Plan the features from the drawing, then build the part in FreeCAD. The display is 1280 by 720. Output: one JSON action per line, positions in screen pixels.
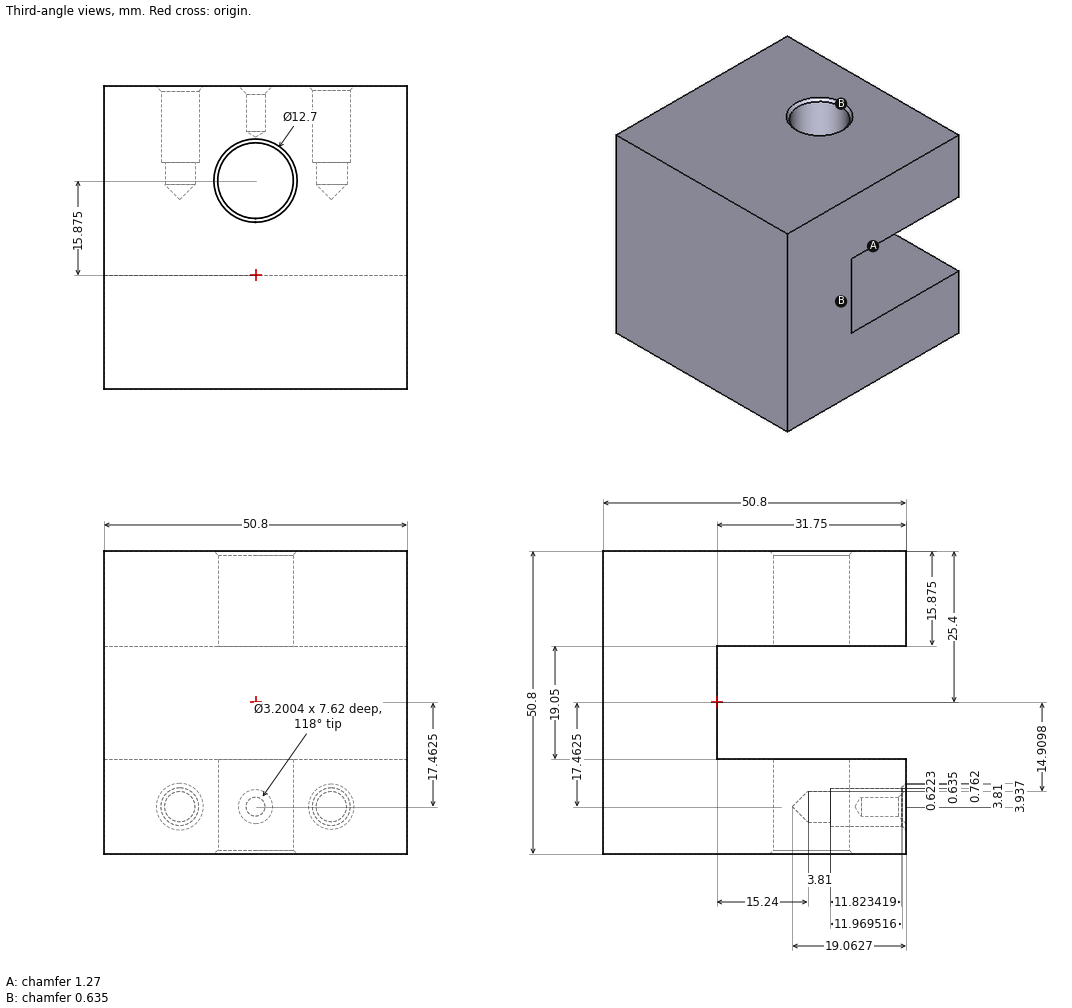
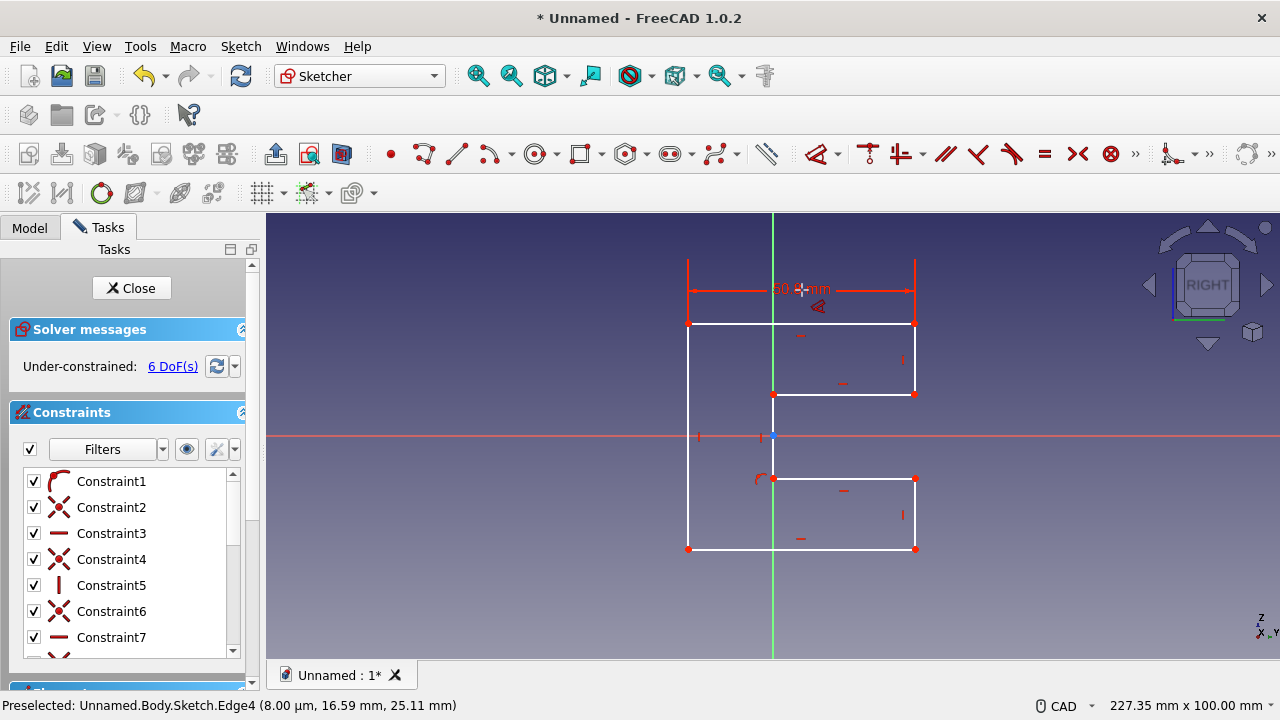
{"action": "left_click", "coordinate": [688, 392]}
{"action": "left_click", "coordinate": [654, 385]}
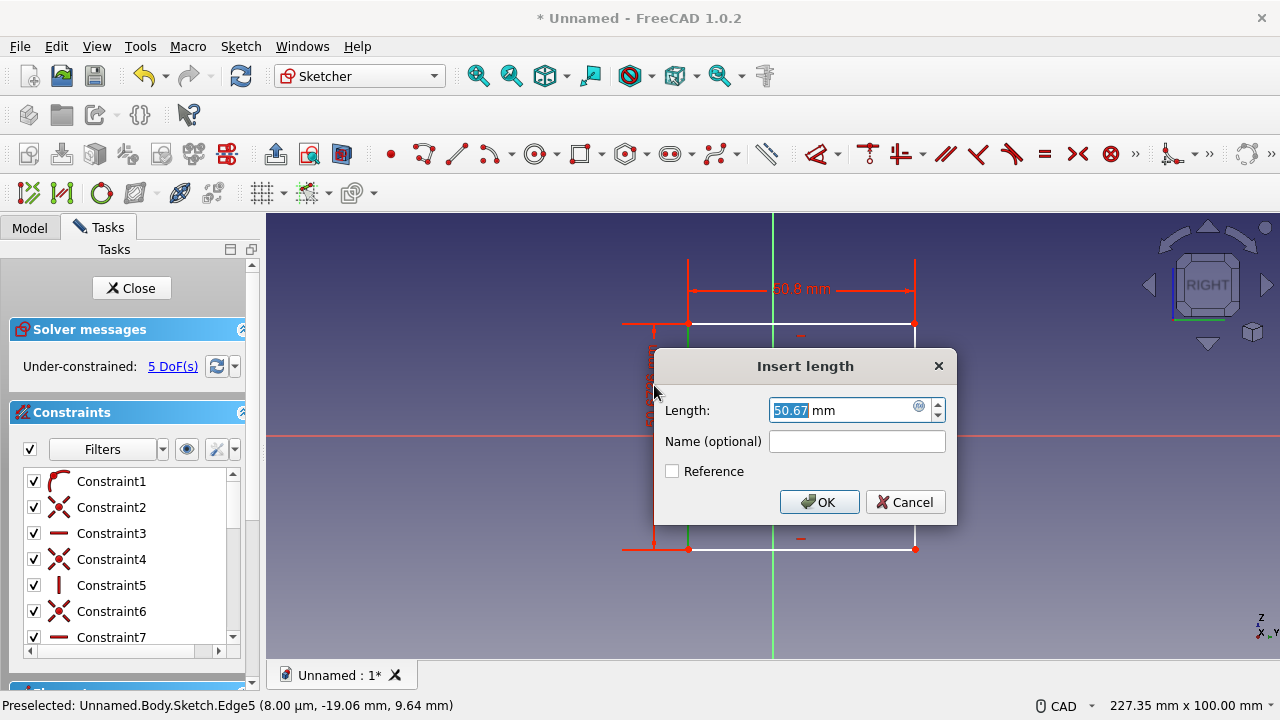
{"action": "type", "text": "50.8"}
{"action": "key", "text": "Return"}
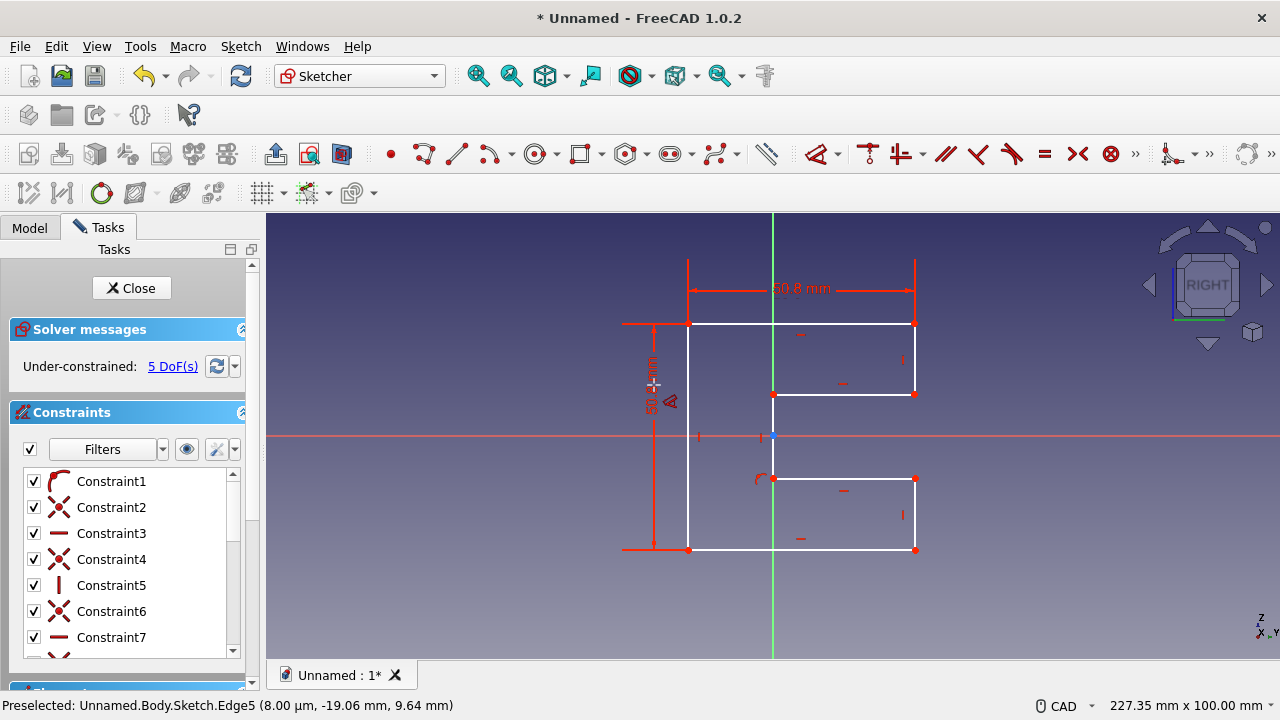
{"action": "left_click", "coordinate": [756, 550]}
{"action": "left_click", "coordinate": [802, 584]}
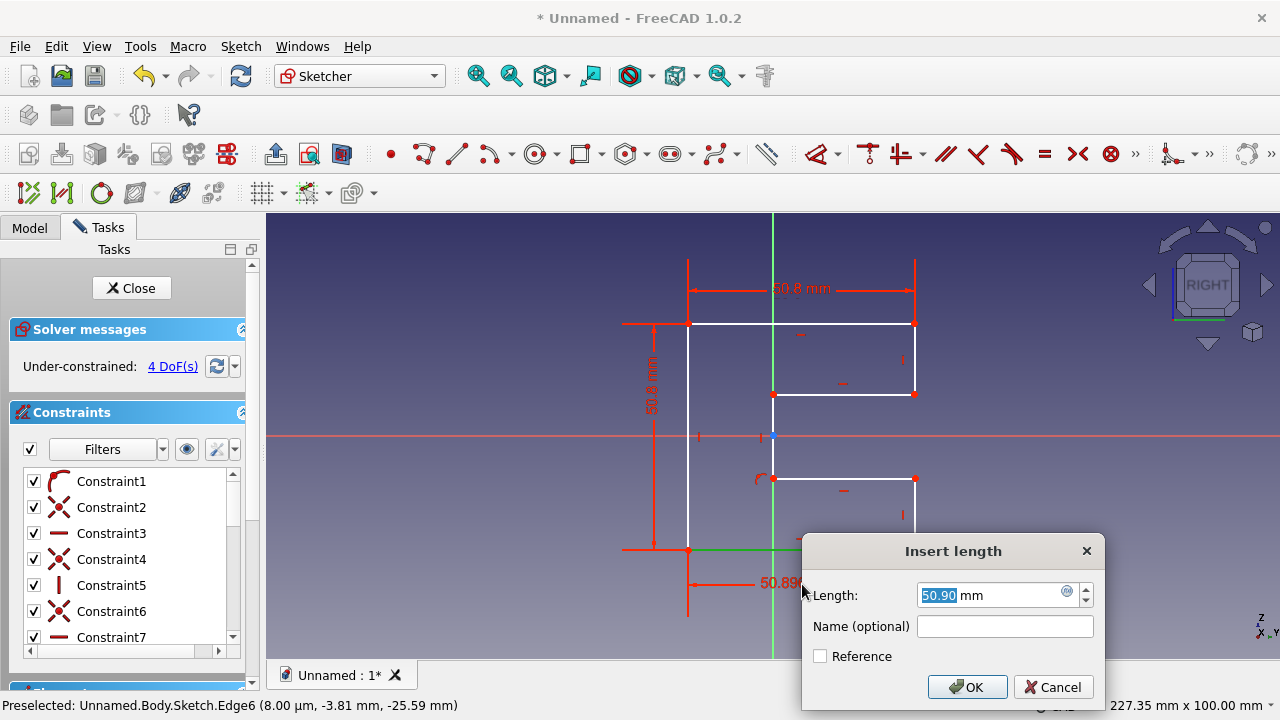
{"action": "type", "text": "50.8"}
{"action": "key", "text": "Return"}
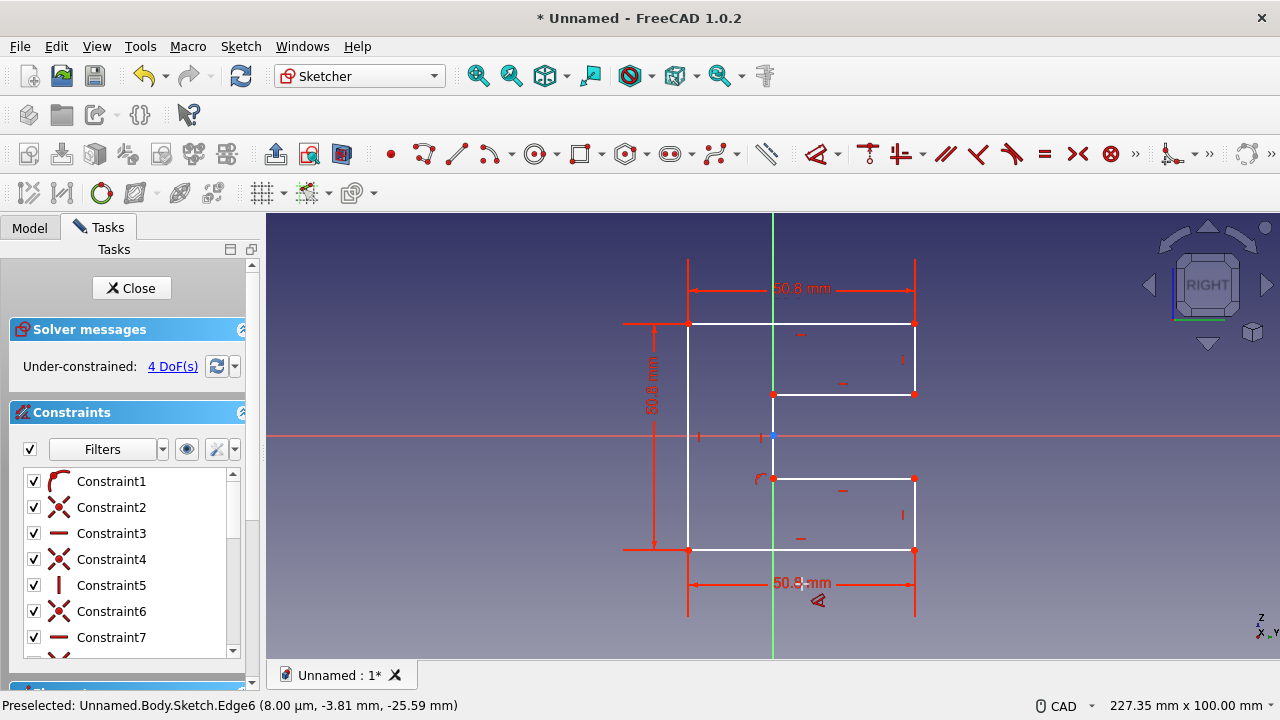
{"action": "left_click", "coordinate": [773, 454]}
{"action": "left_click", "coordinate": [739, 418]}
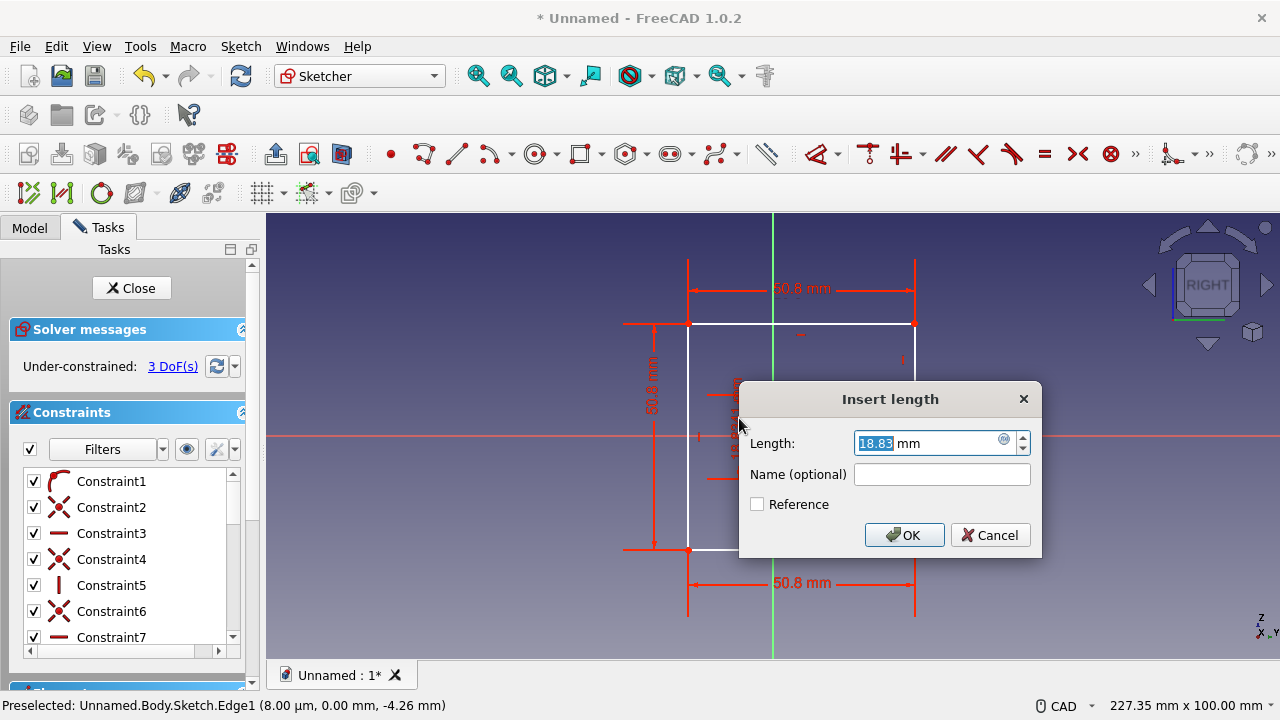
{"action": "type", "text": "19.05"}
{"action": "key", "text": "Return"}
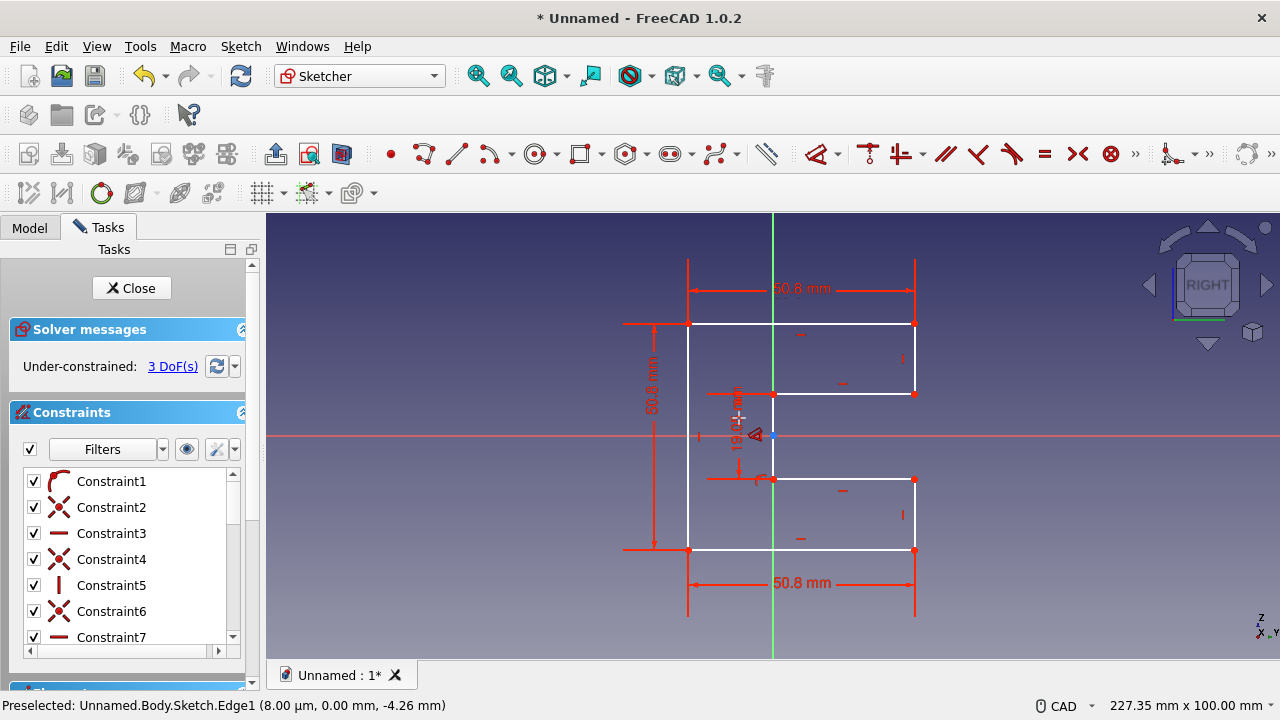
{"action": "left_click", "coordinate": [816, 394]}
{"action": "left_click", "coordinate": [844, 360]}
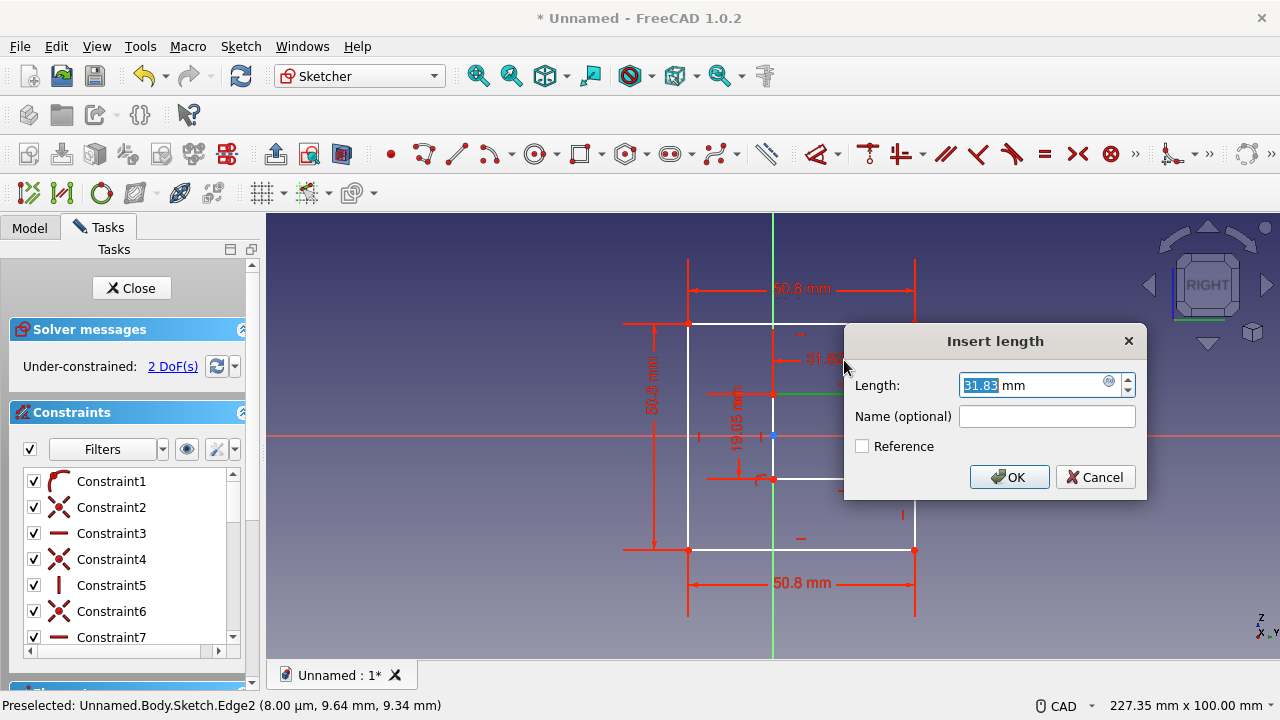
{"action": "type", "text": "31.75"}
{"action": "key", "text": "Return"}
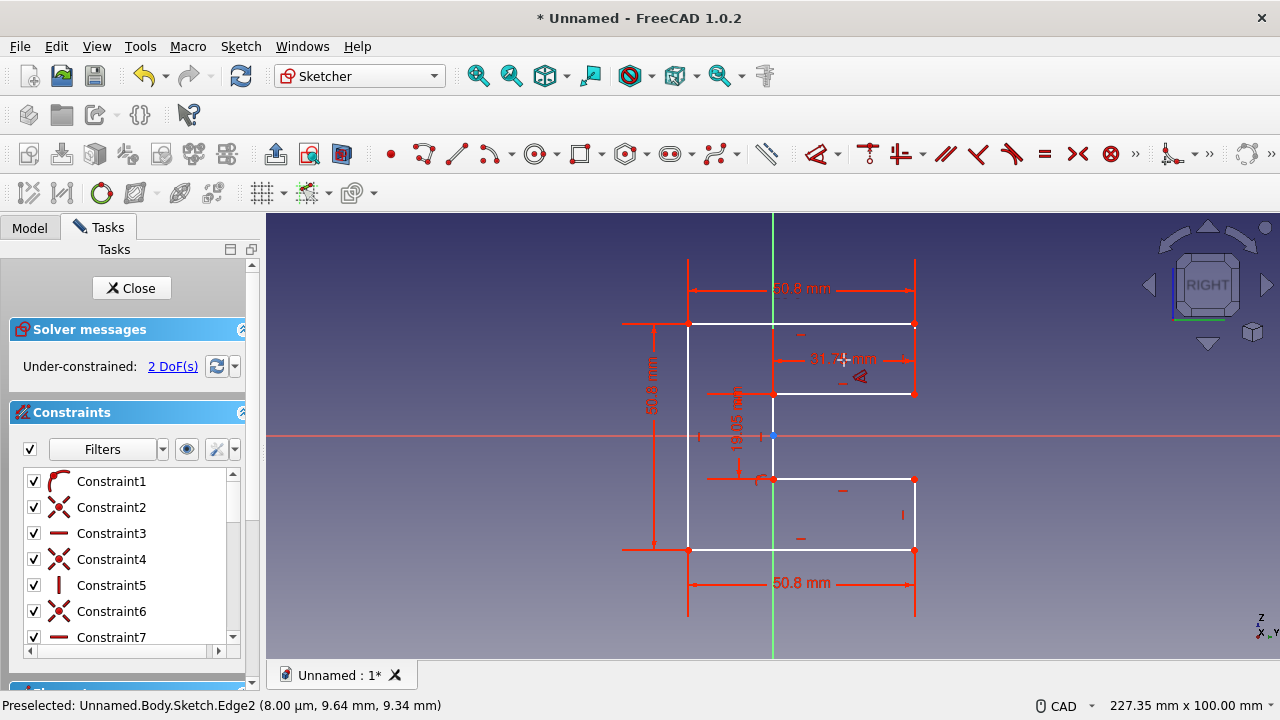
{"action": "left_click", "coordinate": [915, 324]}
{"action": "left_click", "coordinate": [949, 380]}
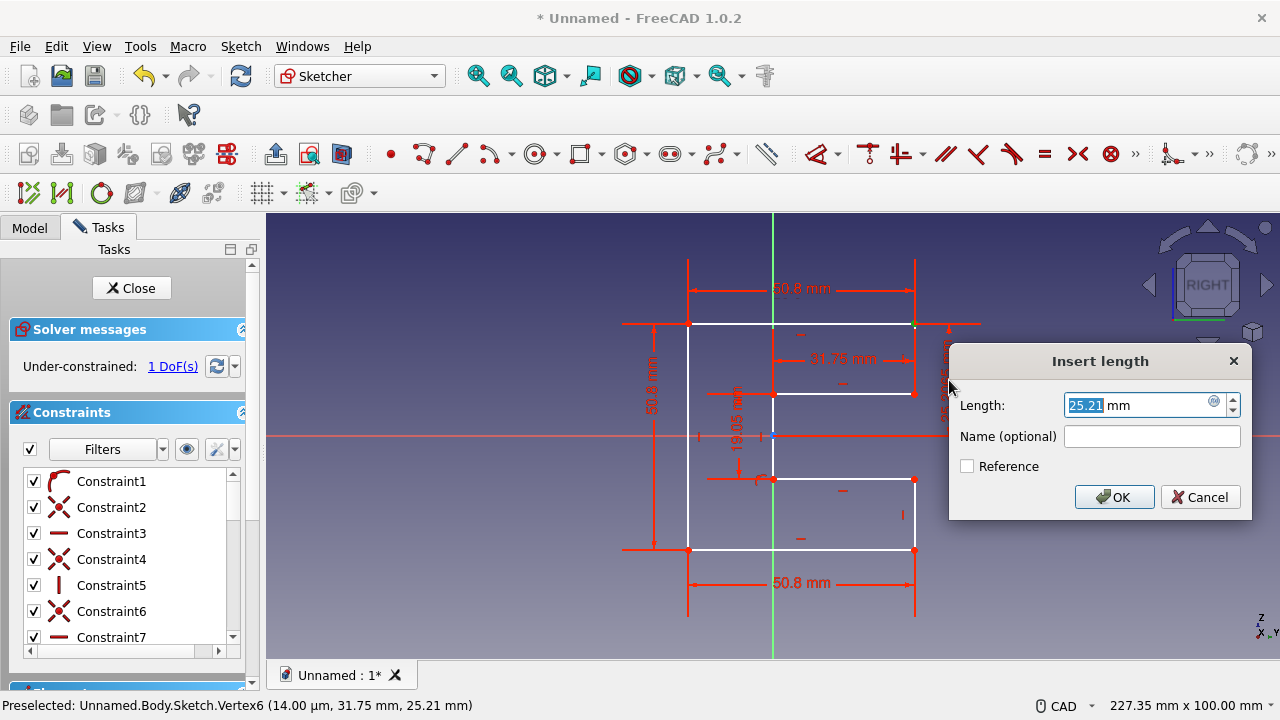
{"action": "type", "text": "25.4"}
{"action": "key", "text": "Return"}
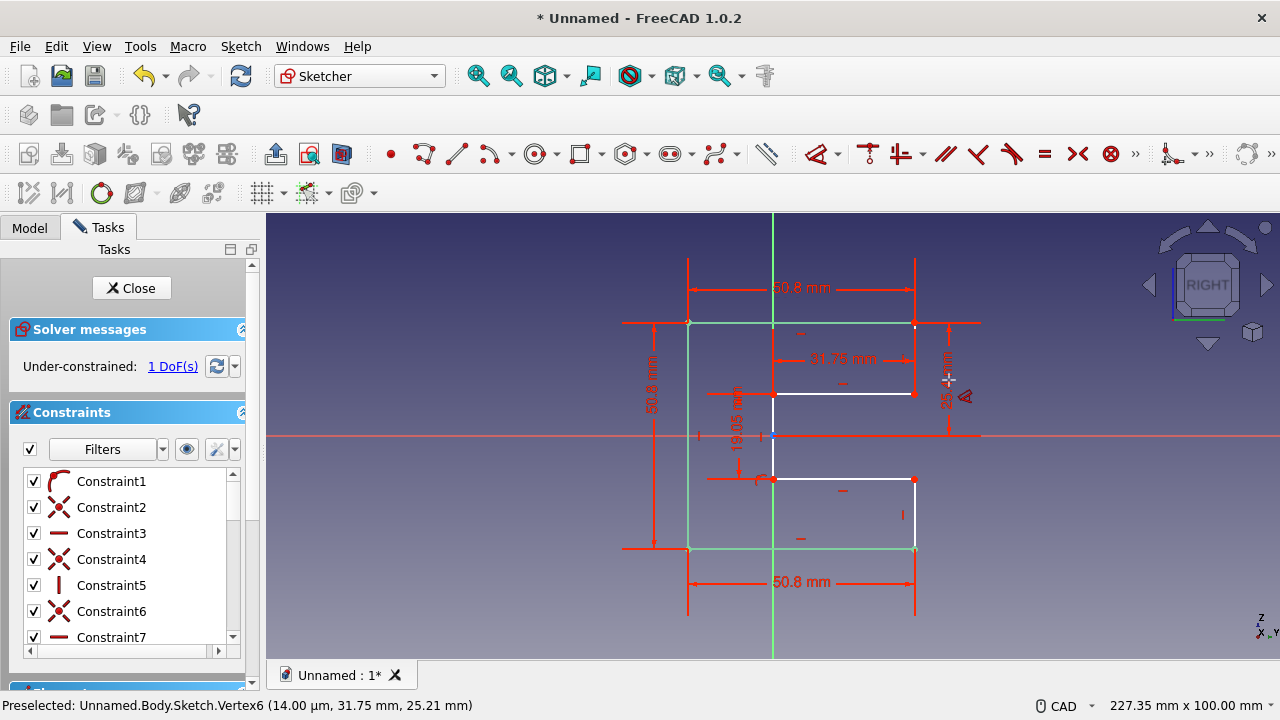
{"action": "left_click", "coordinate": [915, 373]}
{"action": "left_click", "coordinate": [949, 359]}